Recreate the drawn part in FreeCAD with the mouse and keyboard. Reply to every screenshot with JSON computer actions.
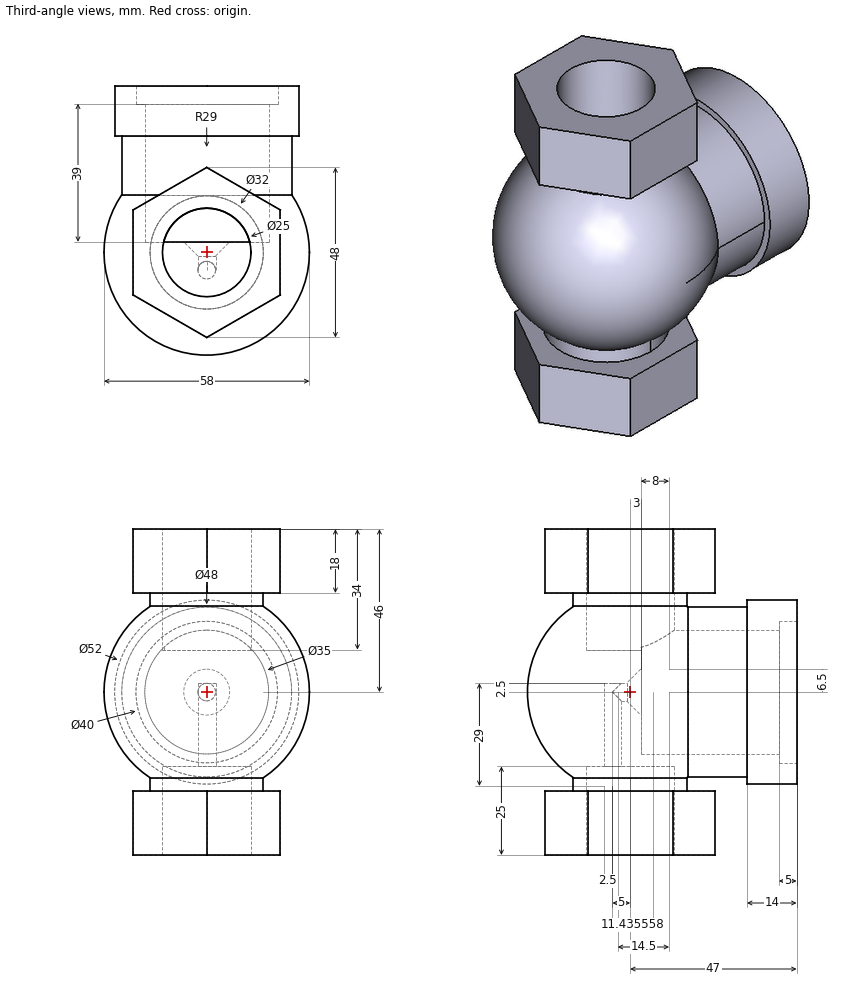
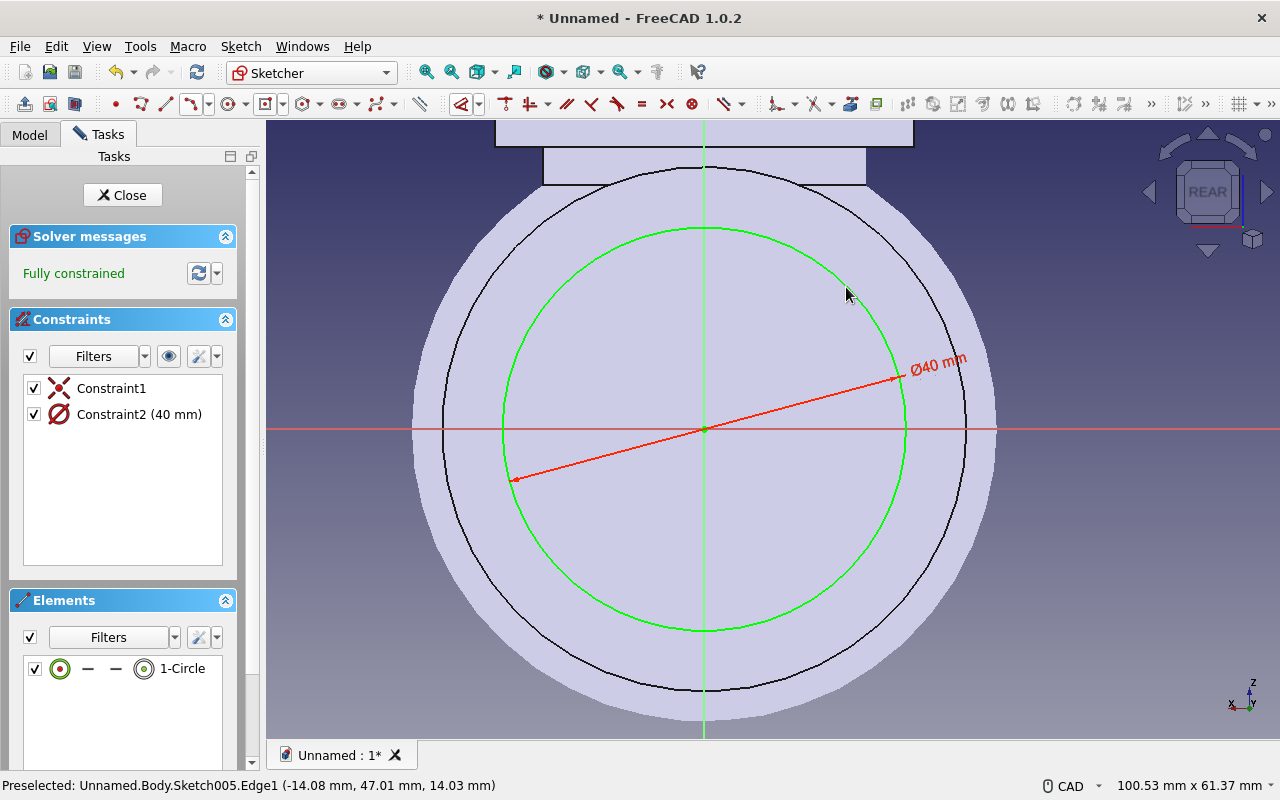
{"action": "left_click", "coordinate": [123, 195]}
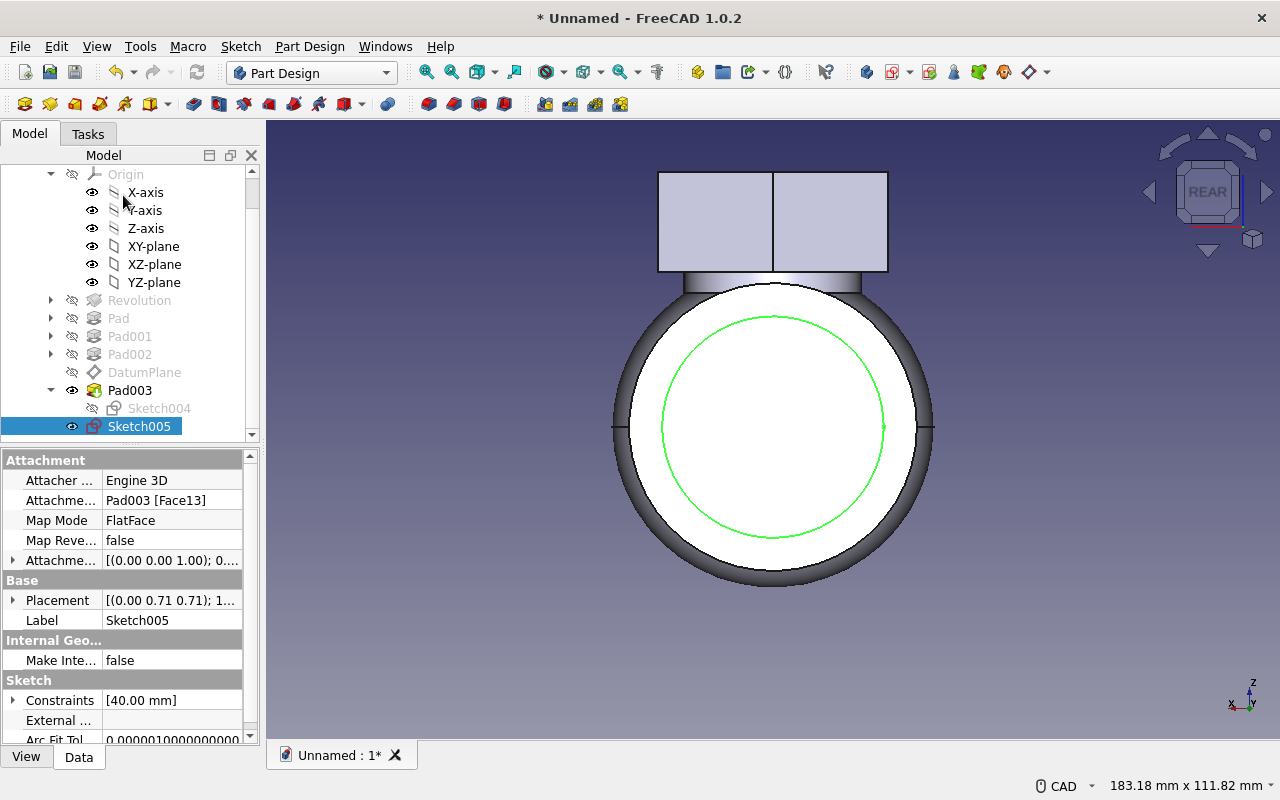
{"action": "left_click", "coordinate": [194, 104]}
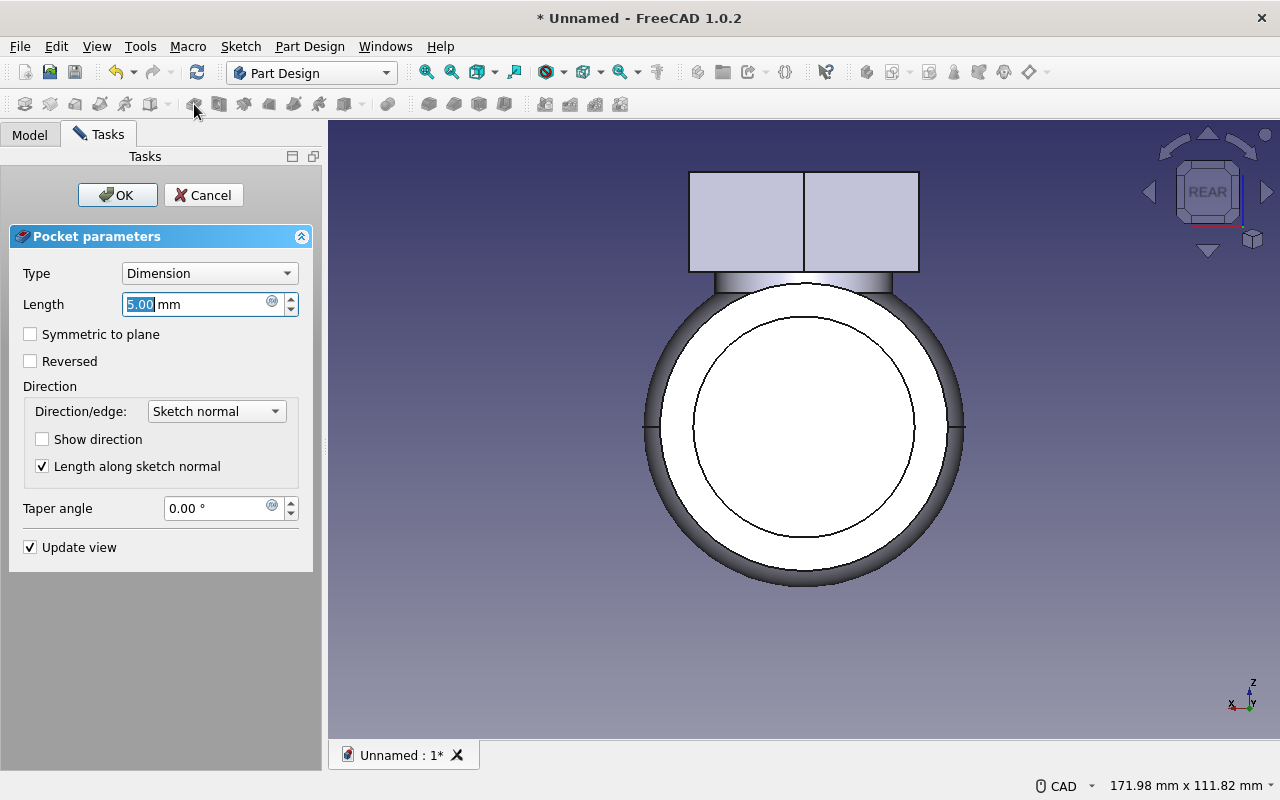
{"action": "type", "text": "5"}
{"action": "key", "text": "Tab"}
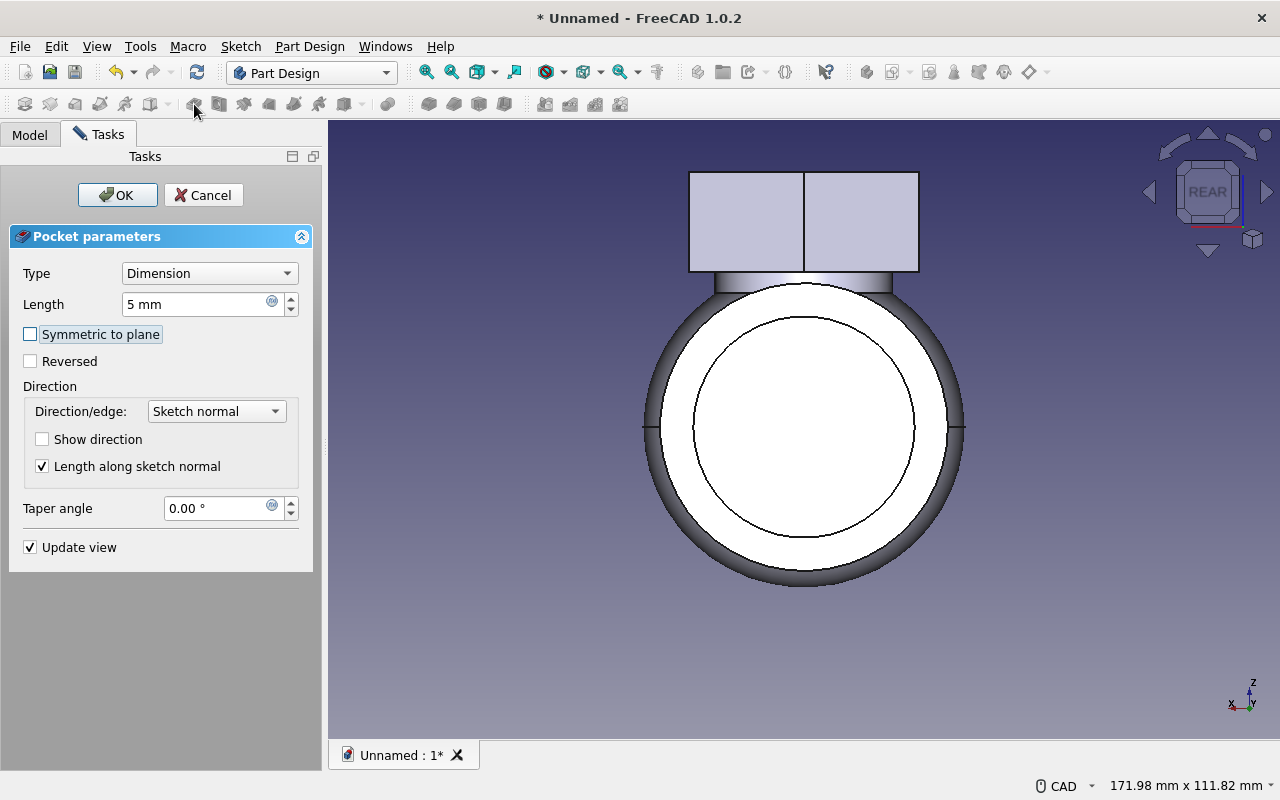
{"action": "left_click", "coordinate": [118, 195]}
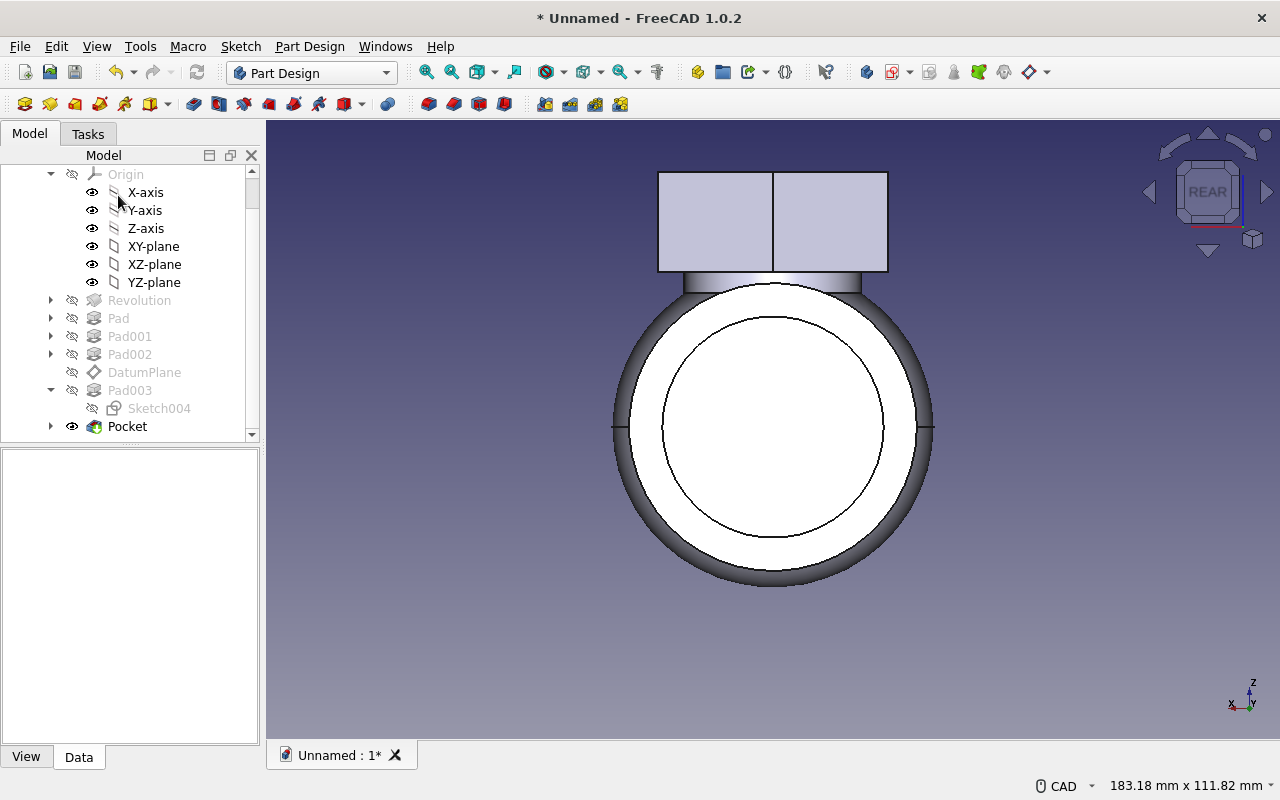
{"action": "key", "text": "0"}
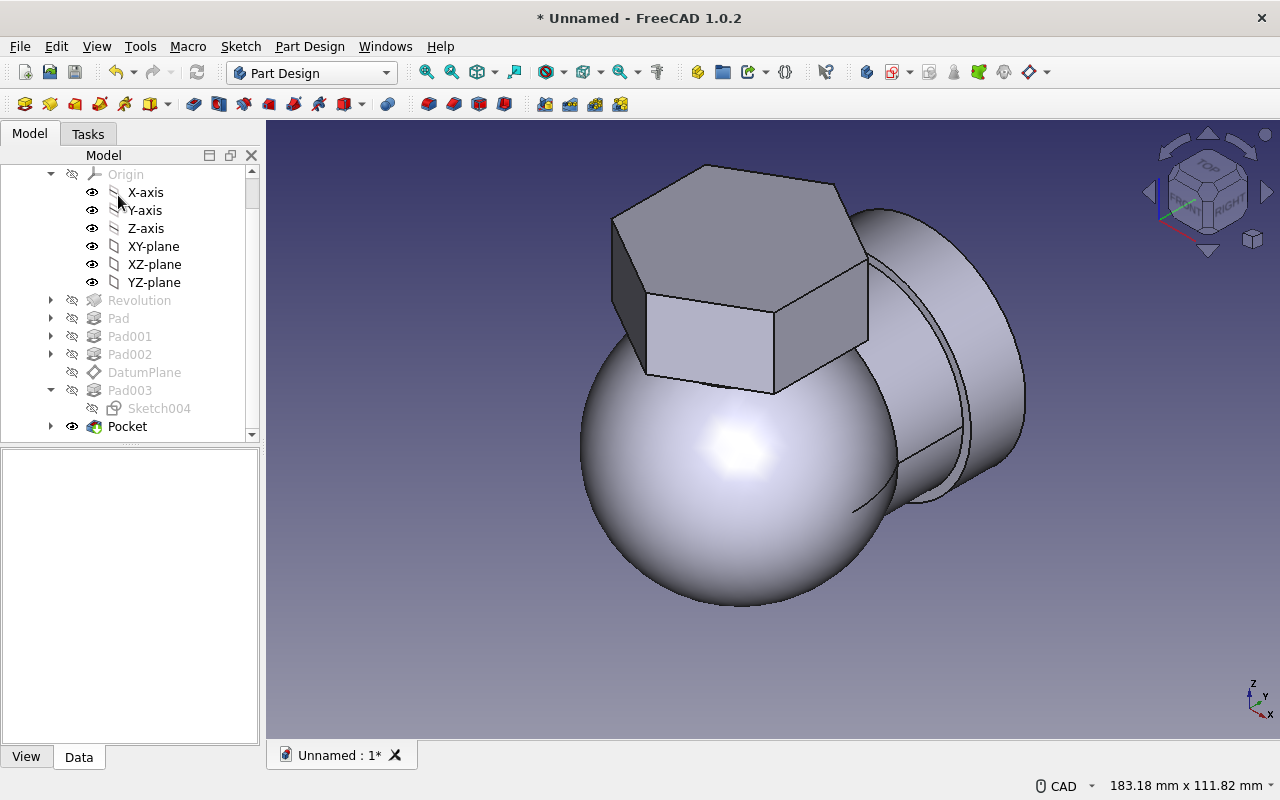
{"action": "left_click", "coordinate": [427, 72]}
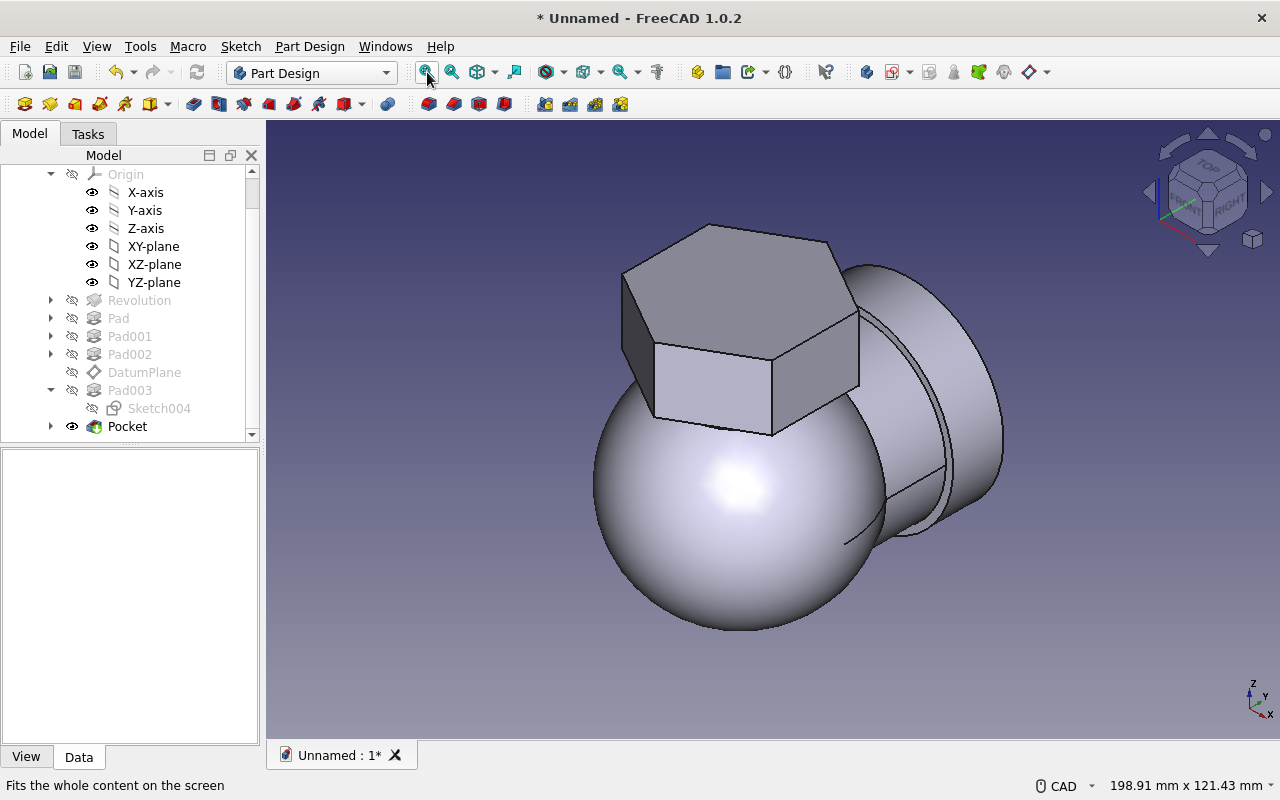
{"action": "left_click", "coordinate": [740, 291]}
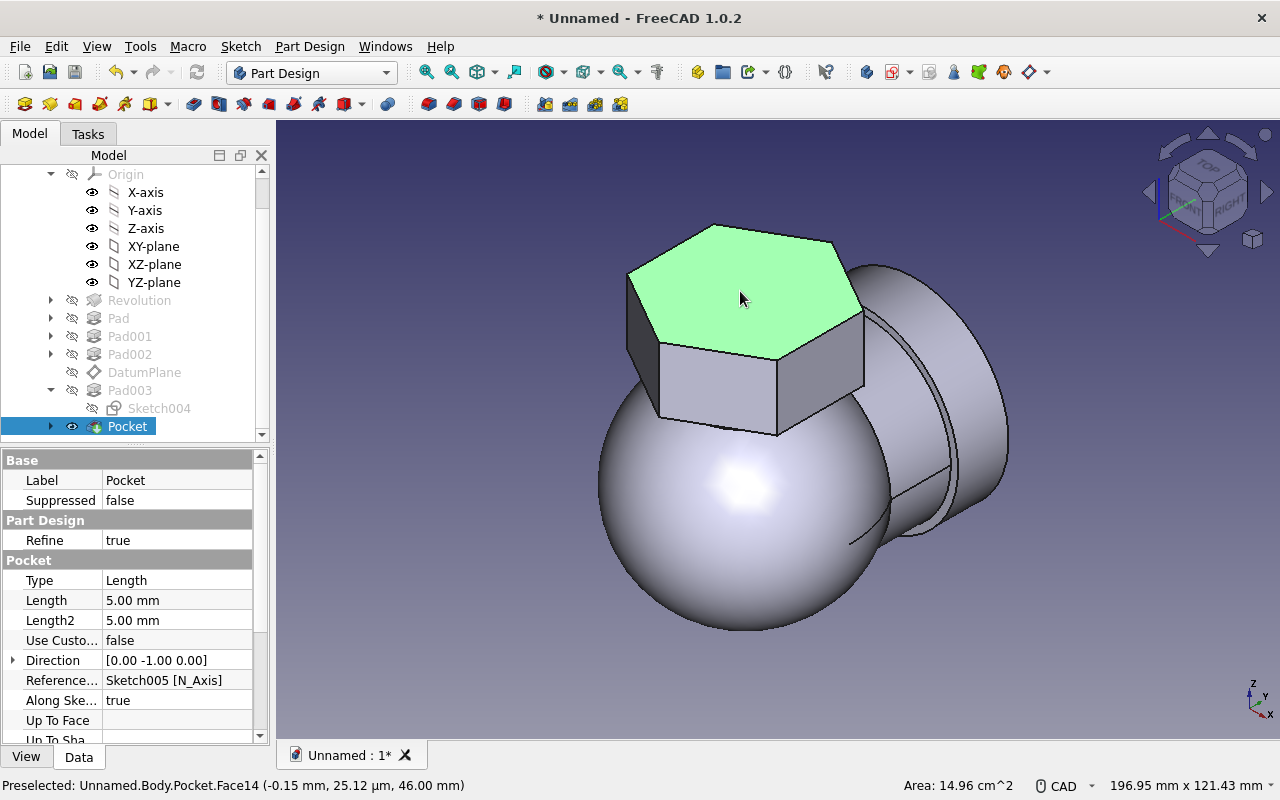
{"action": "left_click", "coordinate": [892, 72]}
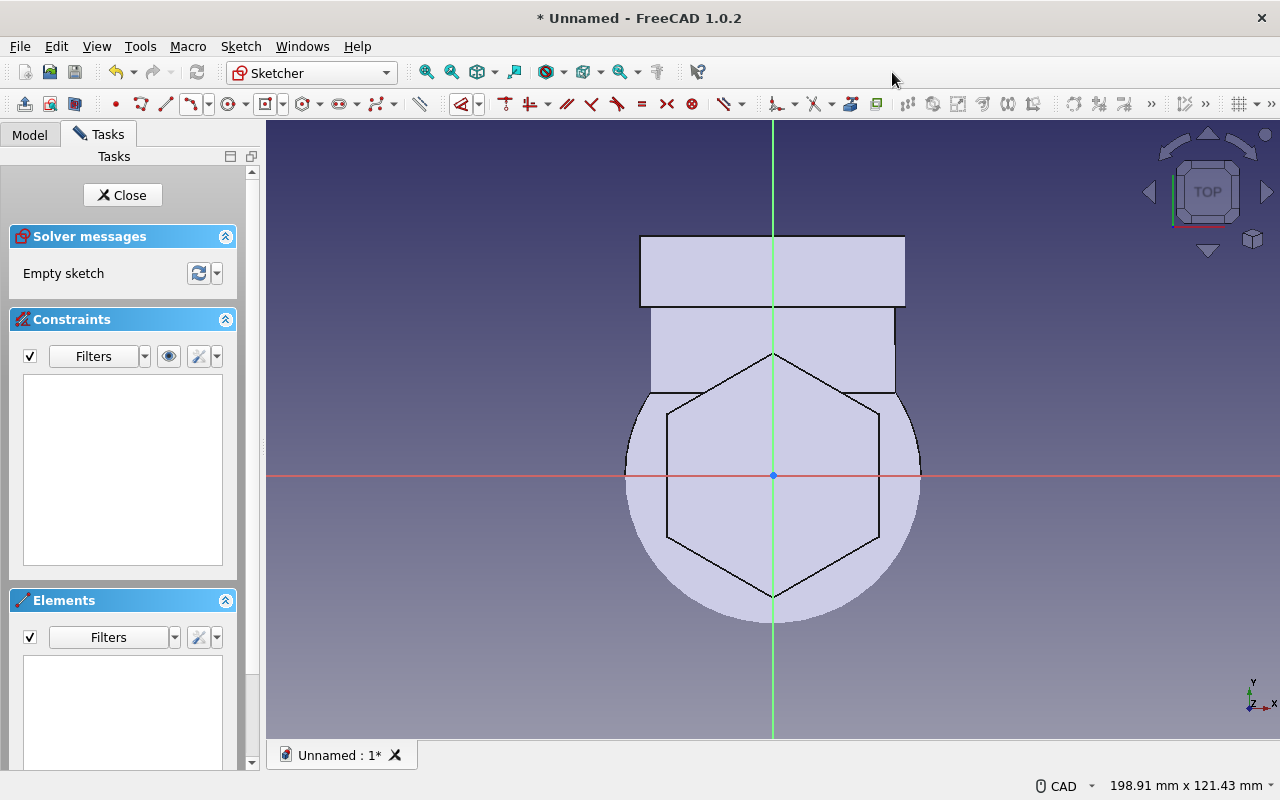
{"action": "scroll", "coordinate": [803, 495], "scroll_direction": "up", "scroll_amount": 6}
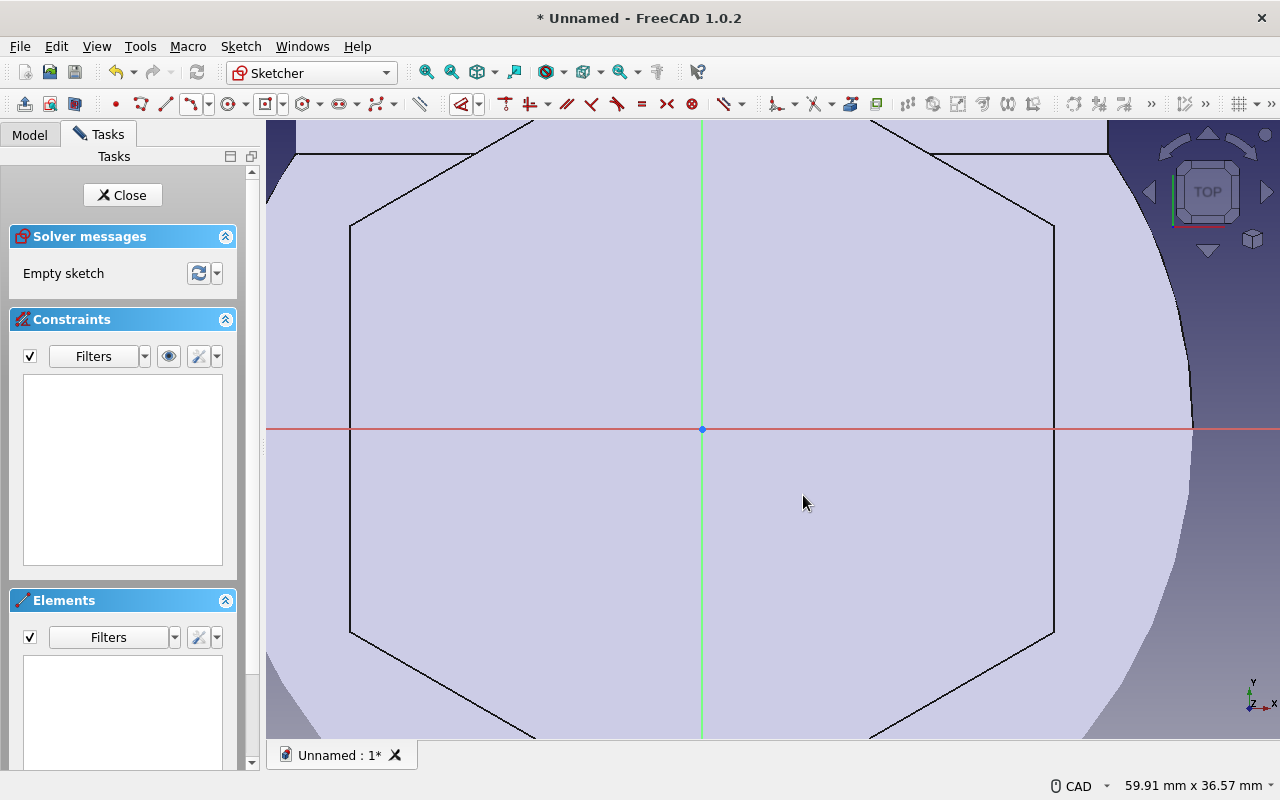
{"action": "left_click", "coordinate": [228, 104]}